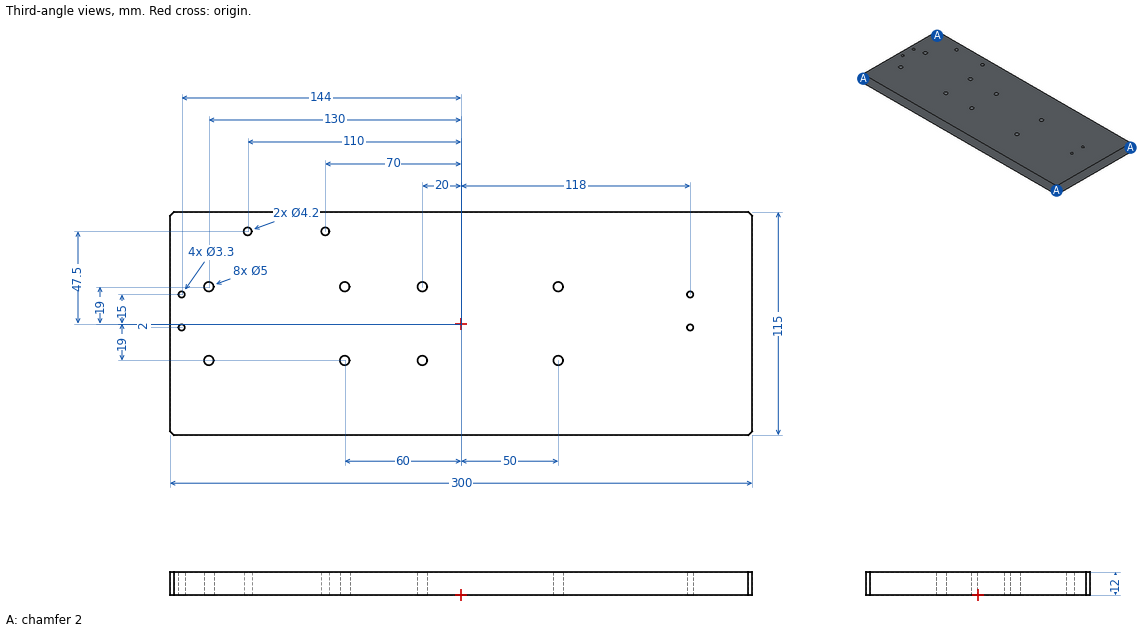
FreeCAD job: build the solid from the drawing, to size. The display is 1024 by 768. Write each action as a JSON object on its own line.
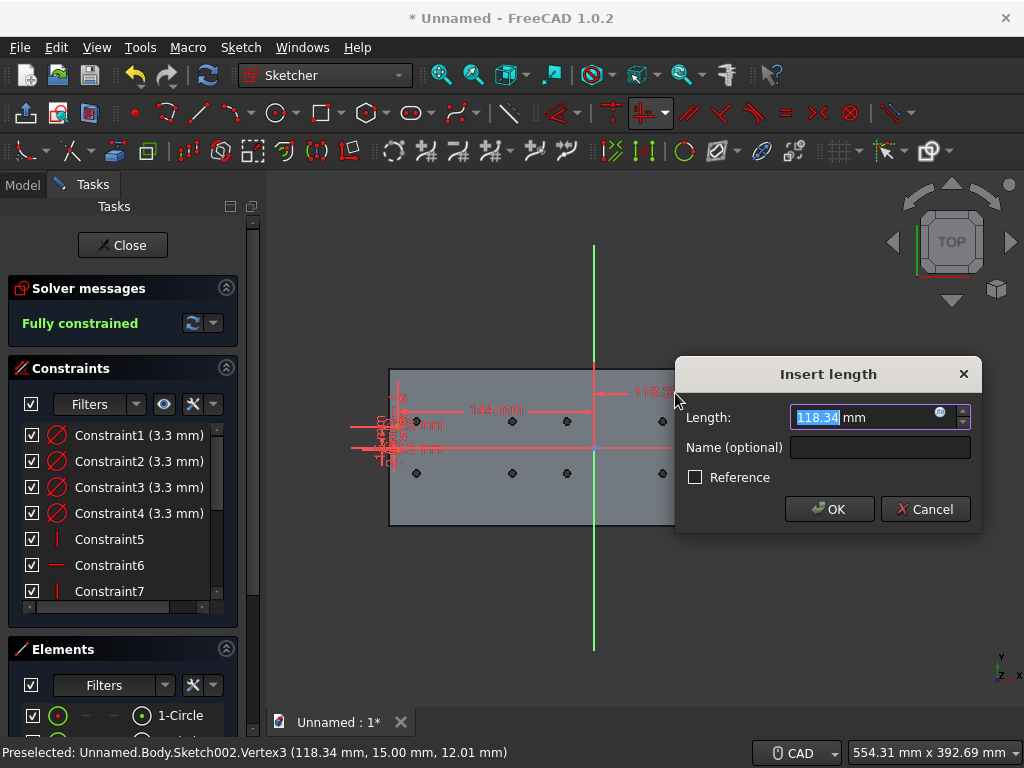
{"action": "type", "text": "118"}
{"action": "key", "text": "Return"}
{"action": "key", "text": "Escape"}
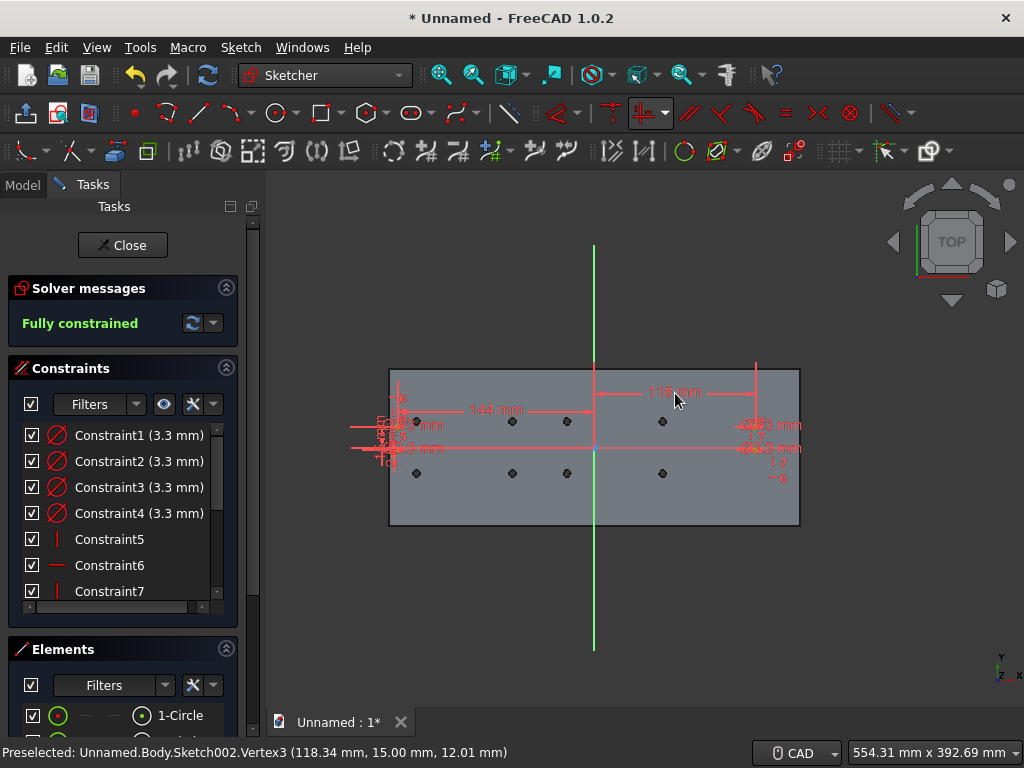
{"action": "left_click", "coordinate": [123, 245]}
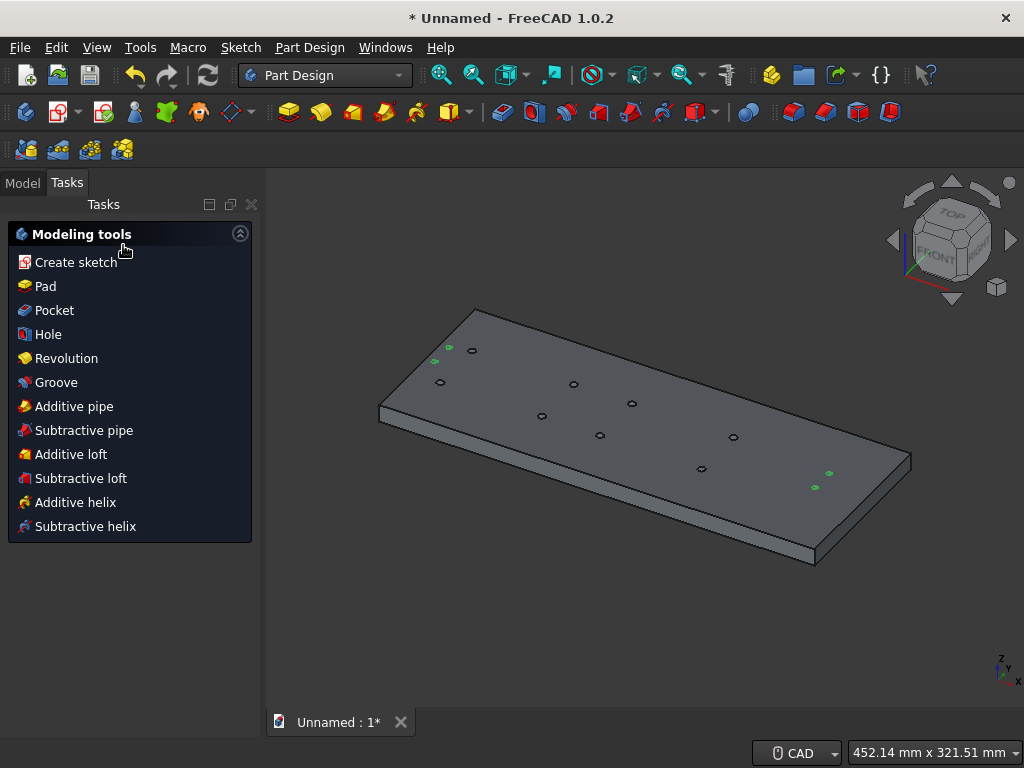
{"action": "left_click", "coordinate": [504, 112]}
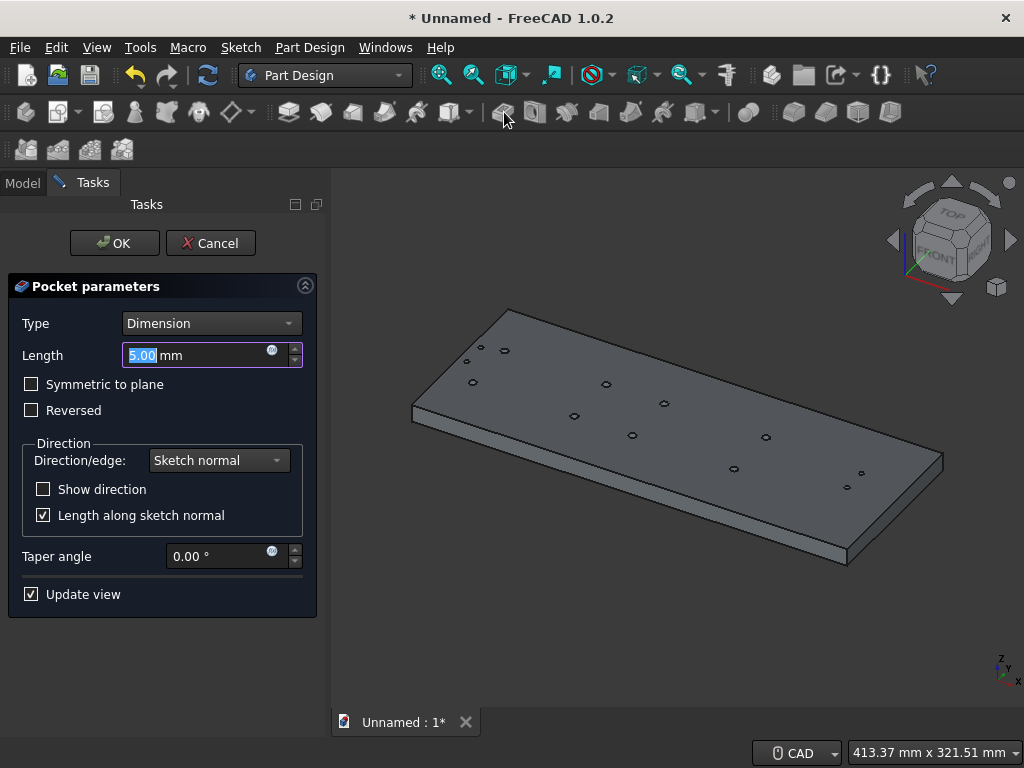
{"action": "left_click", "coordinate": [212, 324]}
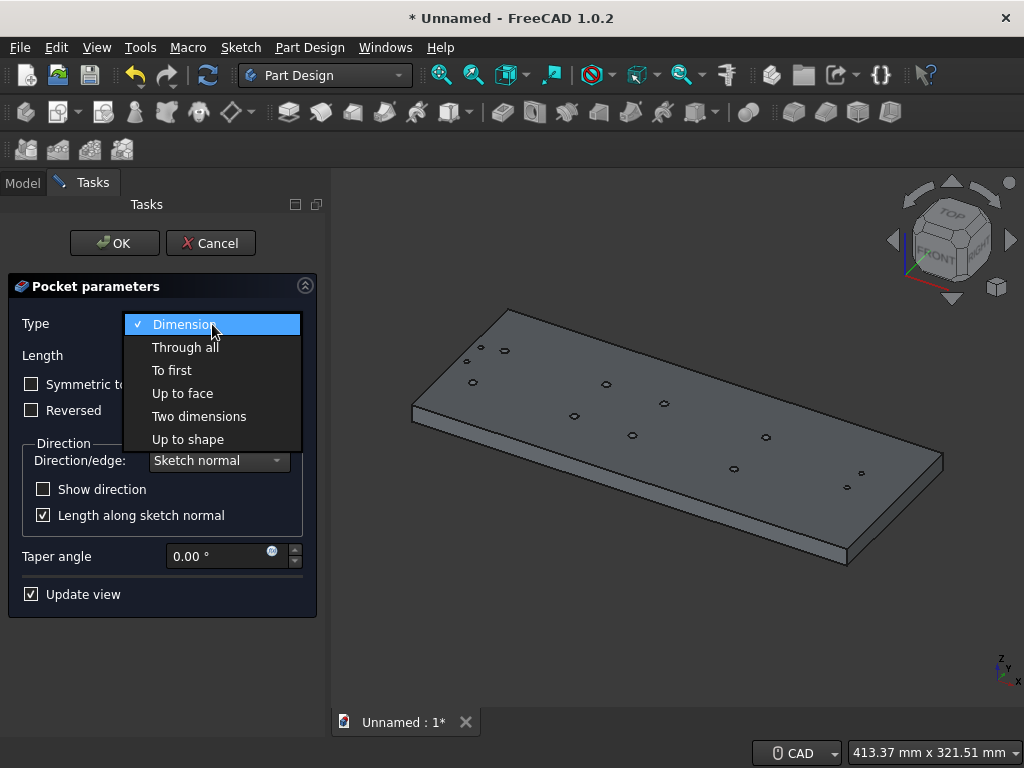
{"action": "left_click", "coordinate": [212, 348]}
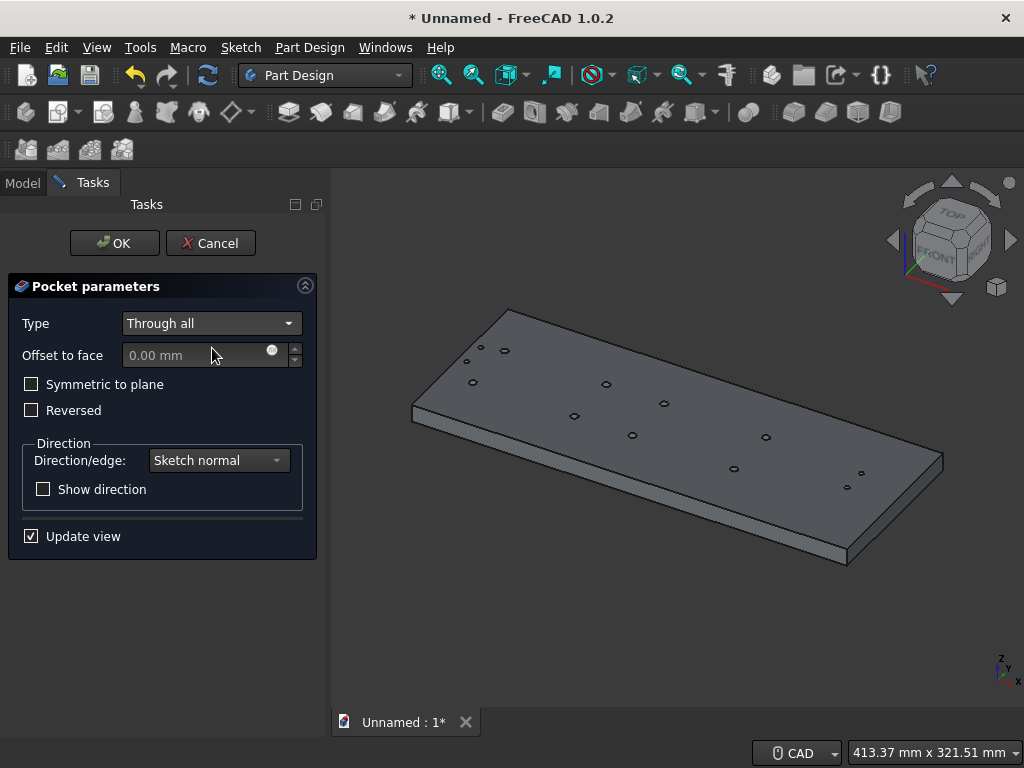
{"action": "left_click", "coordinate": [115, 243]}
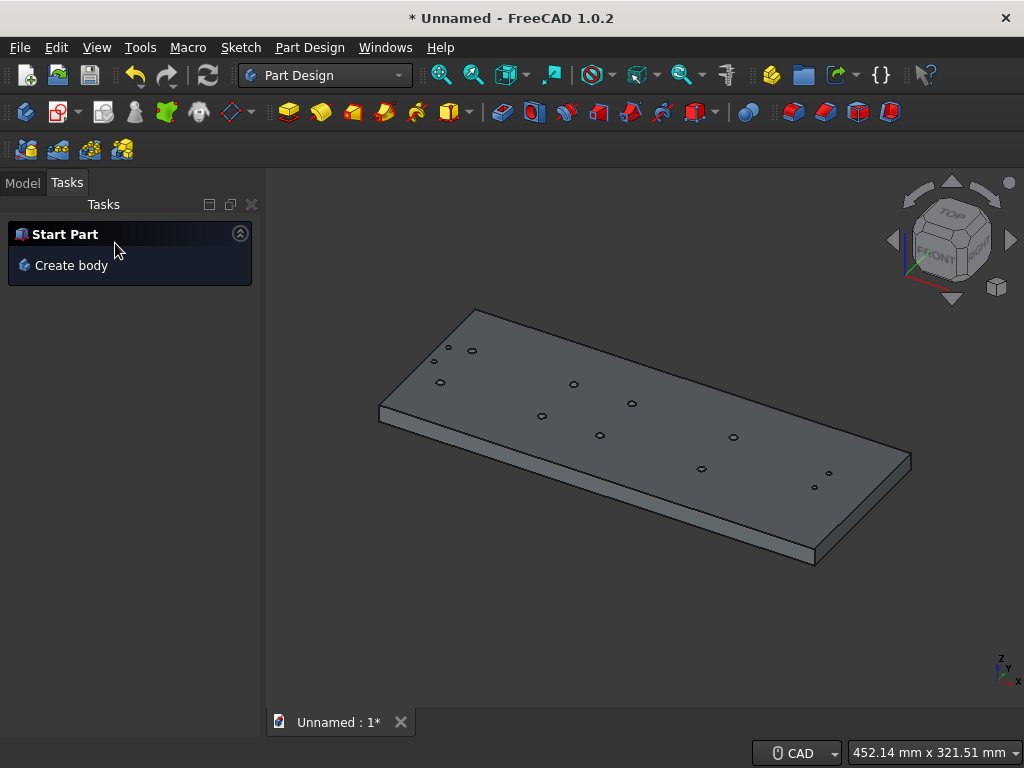
{"action": "key", "text": "5"}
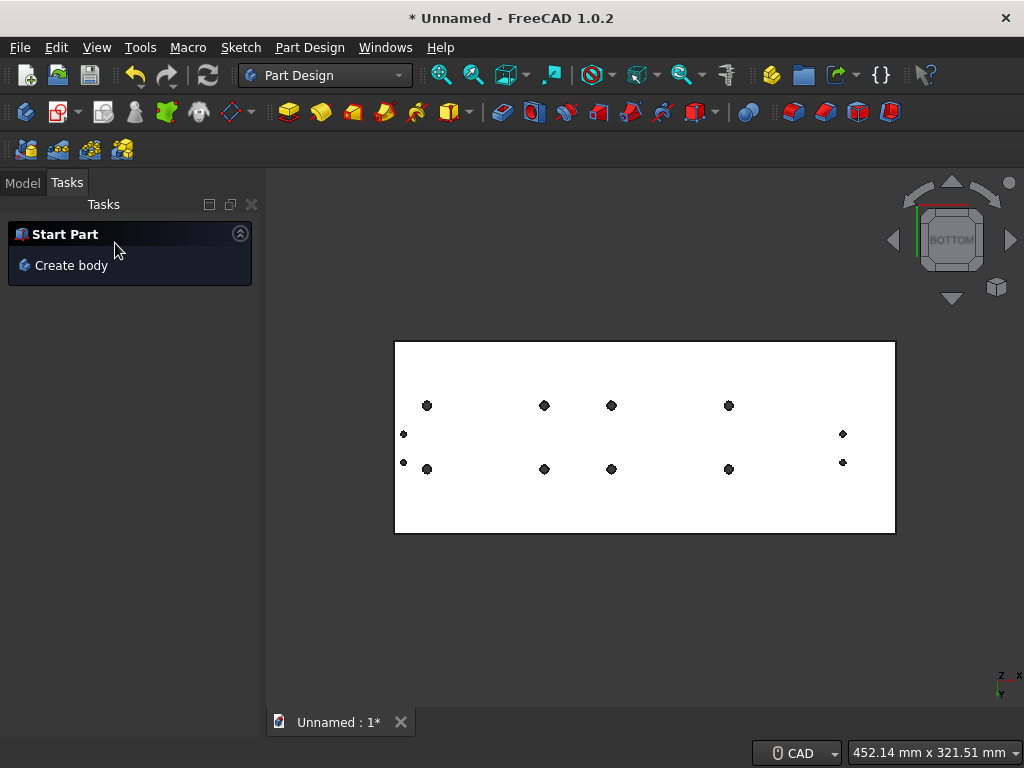
{"action": "left_click", "coordinate": [789, 409]}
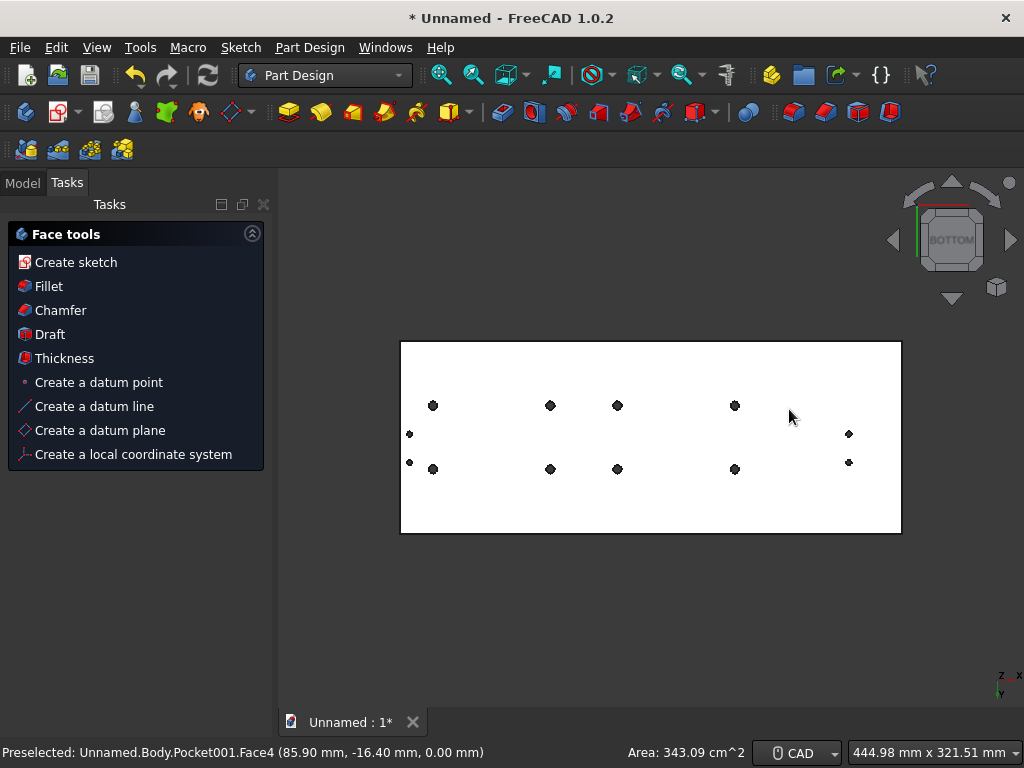
{"action": "left_click", "coordinate": [58, 112]}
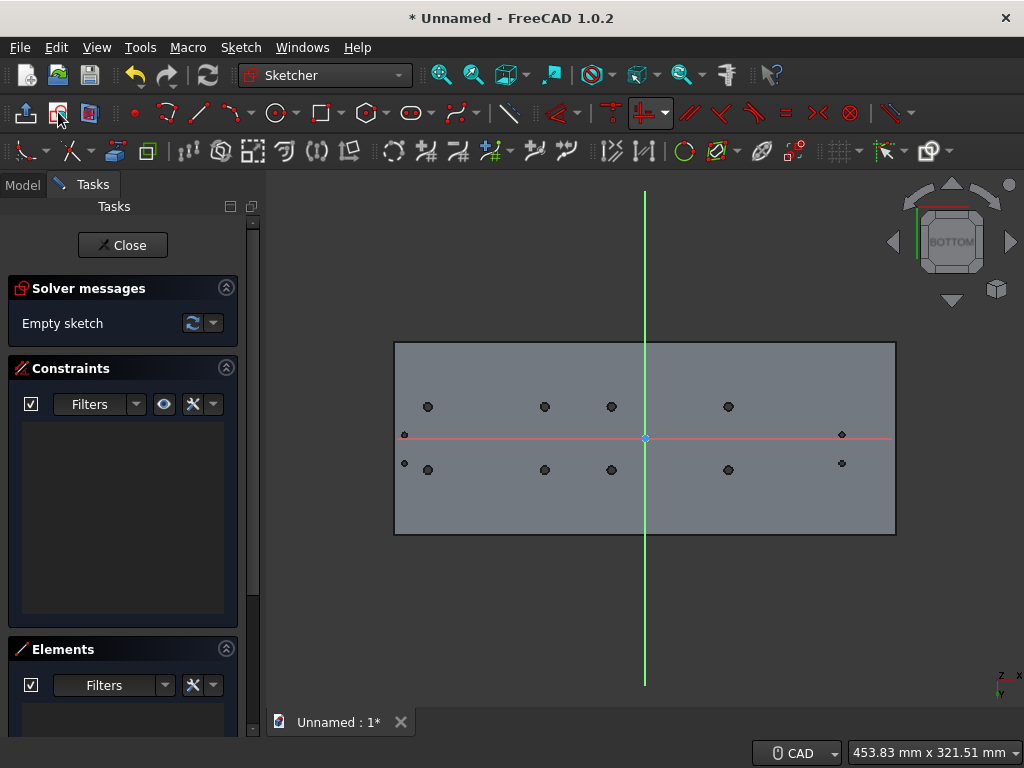
{"action": "scroll", "coordinate": [474, 538], "scroll_direction": "up", "scroll_amount": 8}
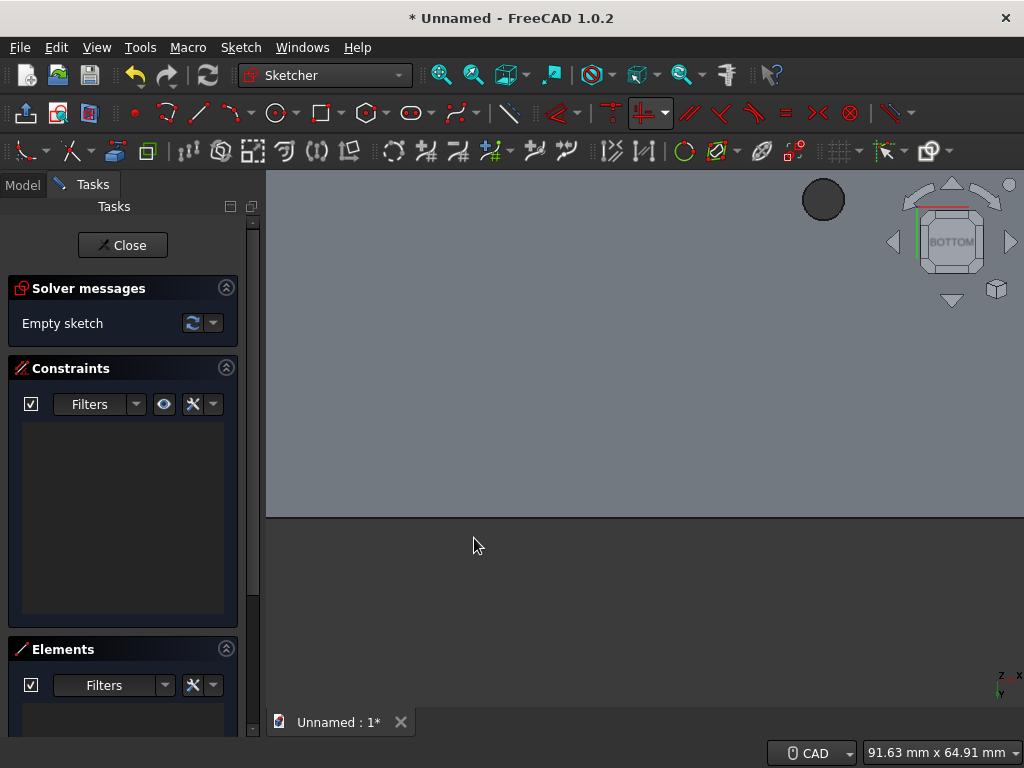
{"action": "left_click", "coordinate": [276, 114]}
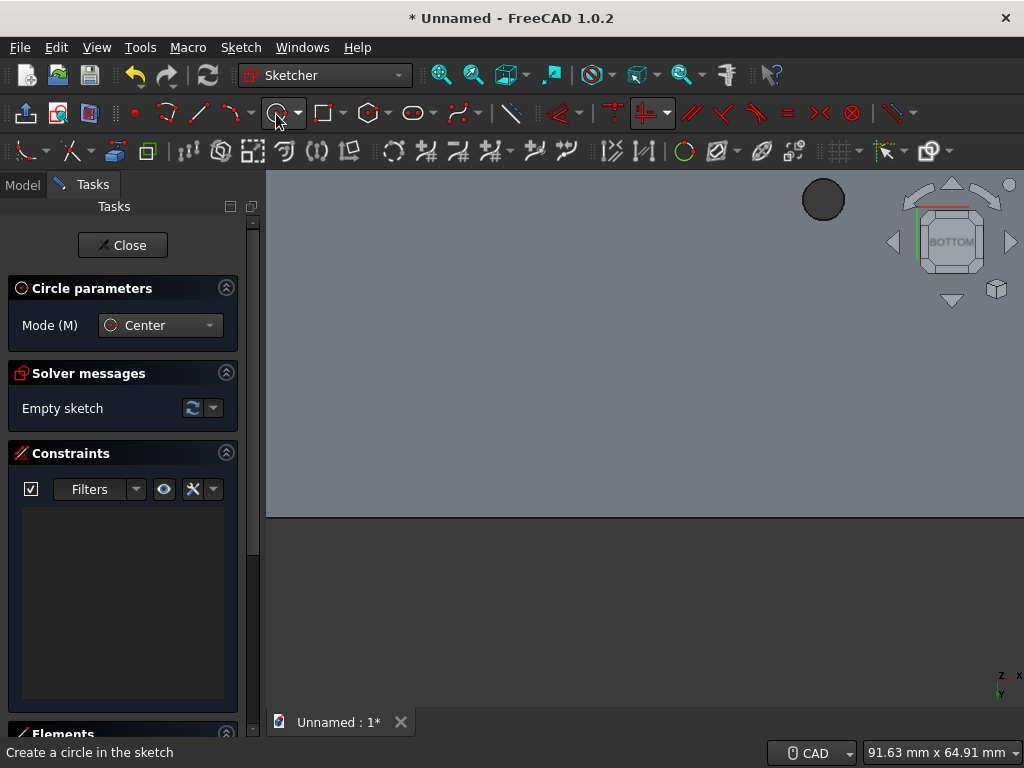
{"action": "scroll", "coordinate": [410, 435], "scroll_direction": "up", "scroll_amount": 2}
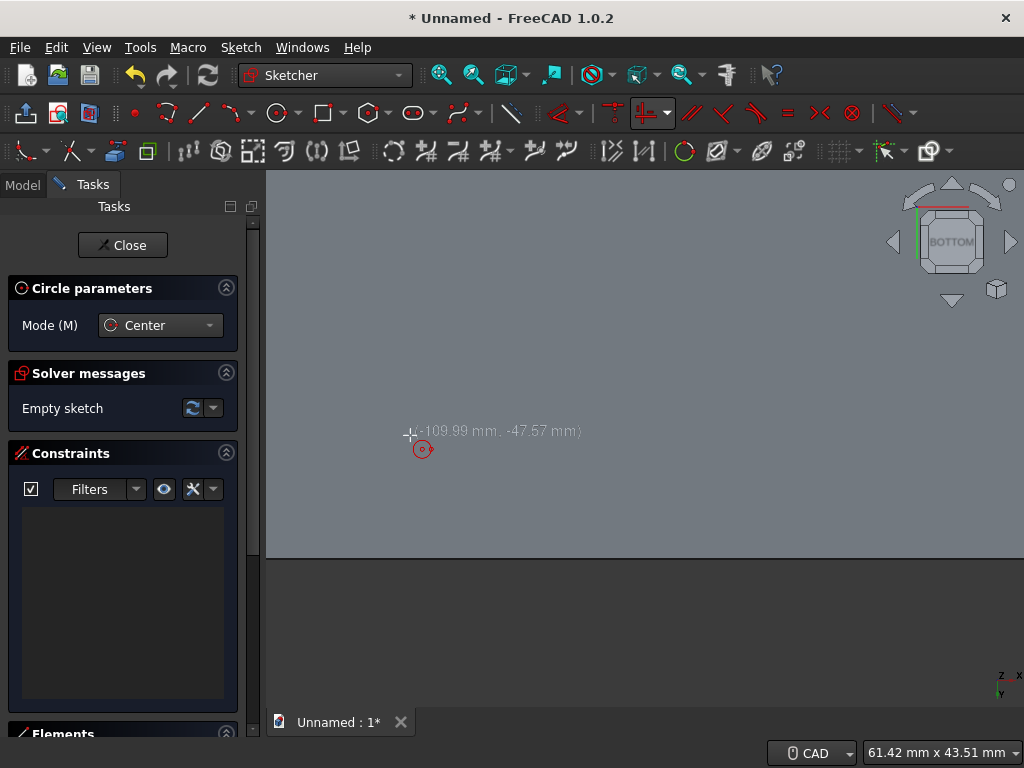
{"action": "left_click", "coordinate": [410, 435]}
{"action": "mouse_move", "coordinate": [428, 417]}